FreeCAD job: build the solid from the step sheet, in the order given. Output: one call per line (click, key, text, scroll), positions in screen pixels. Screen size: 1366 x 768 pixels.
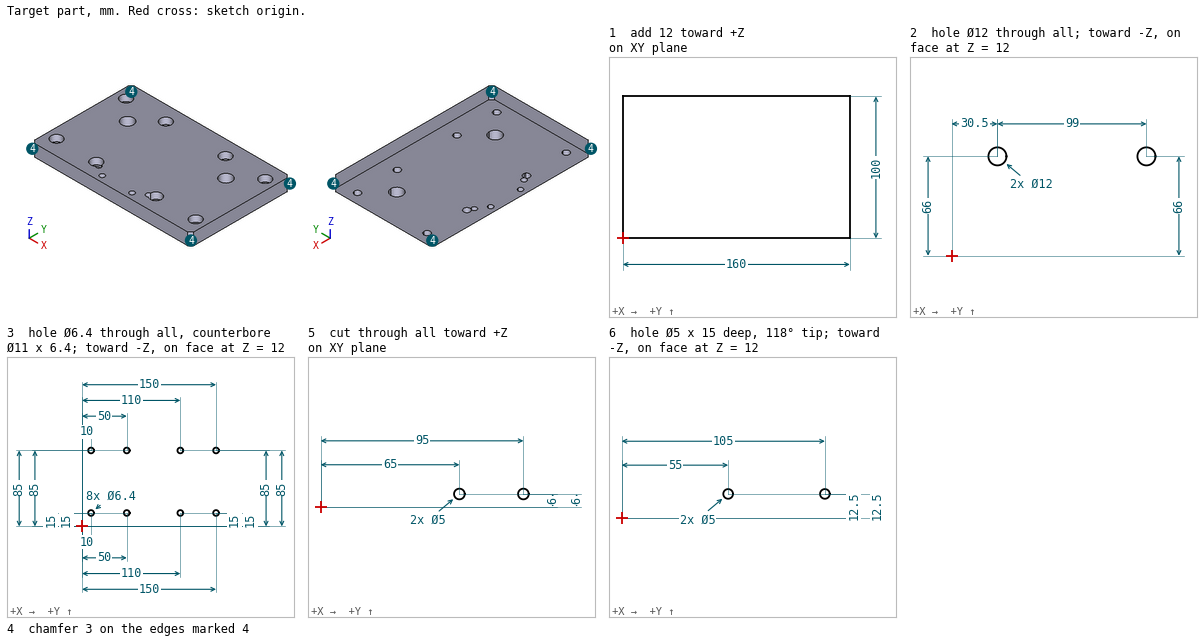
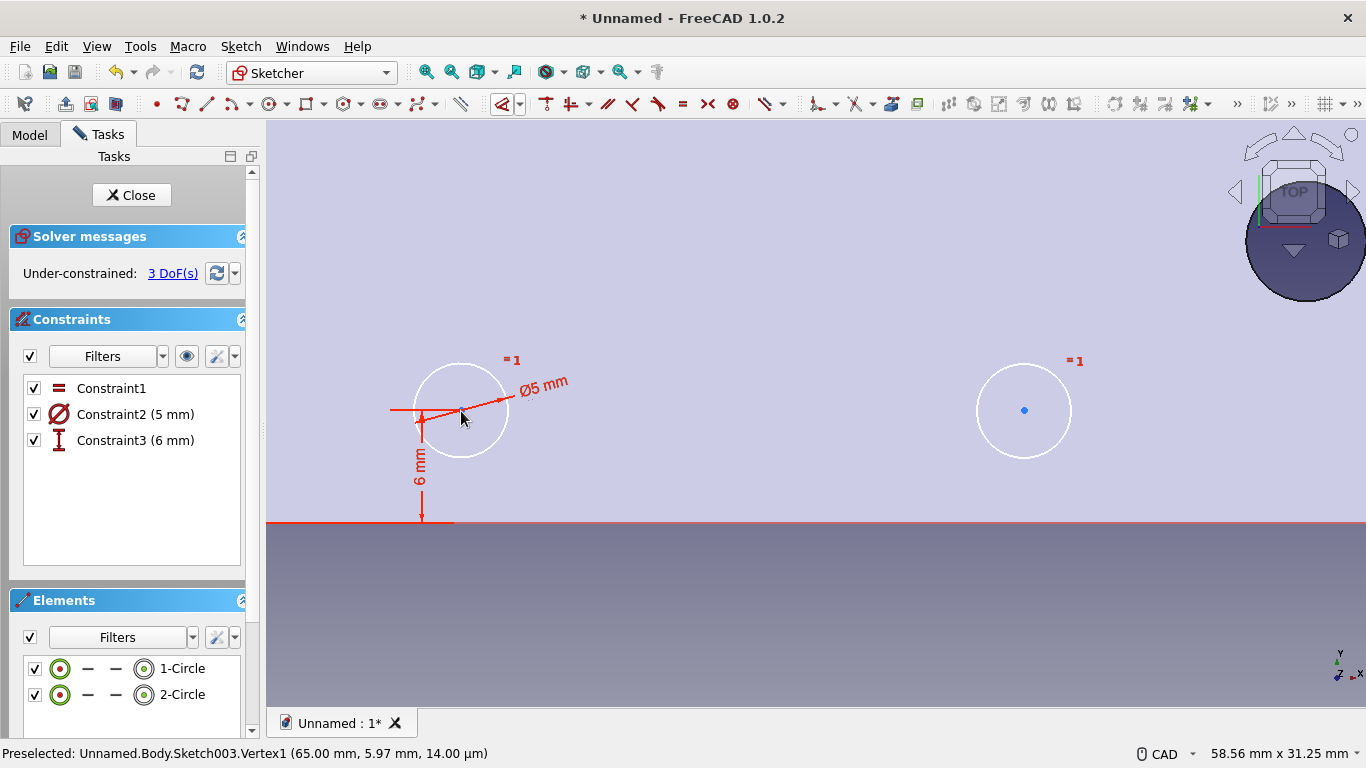
click(1024, 411)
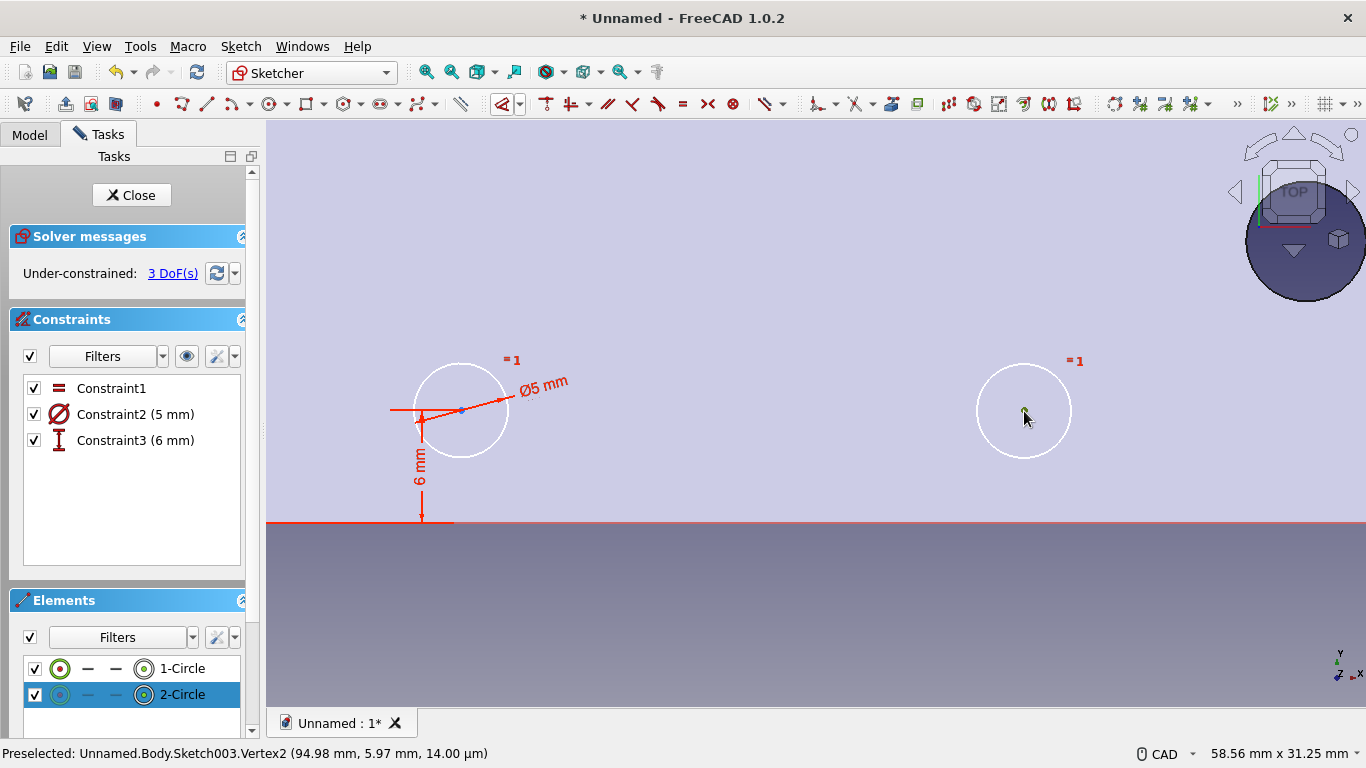
key(i)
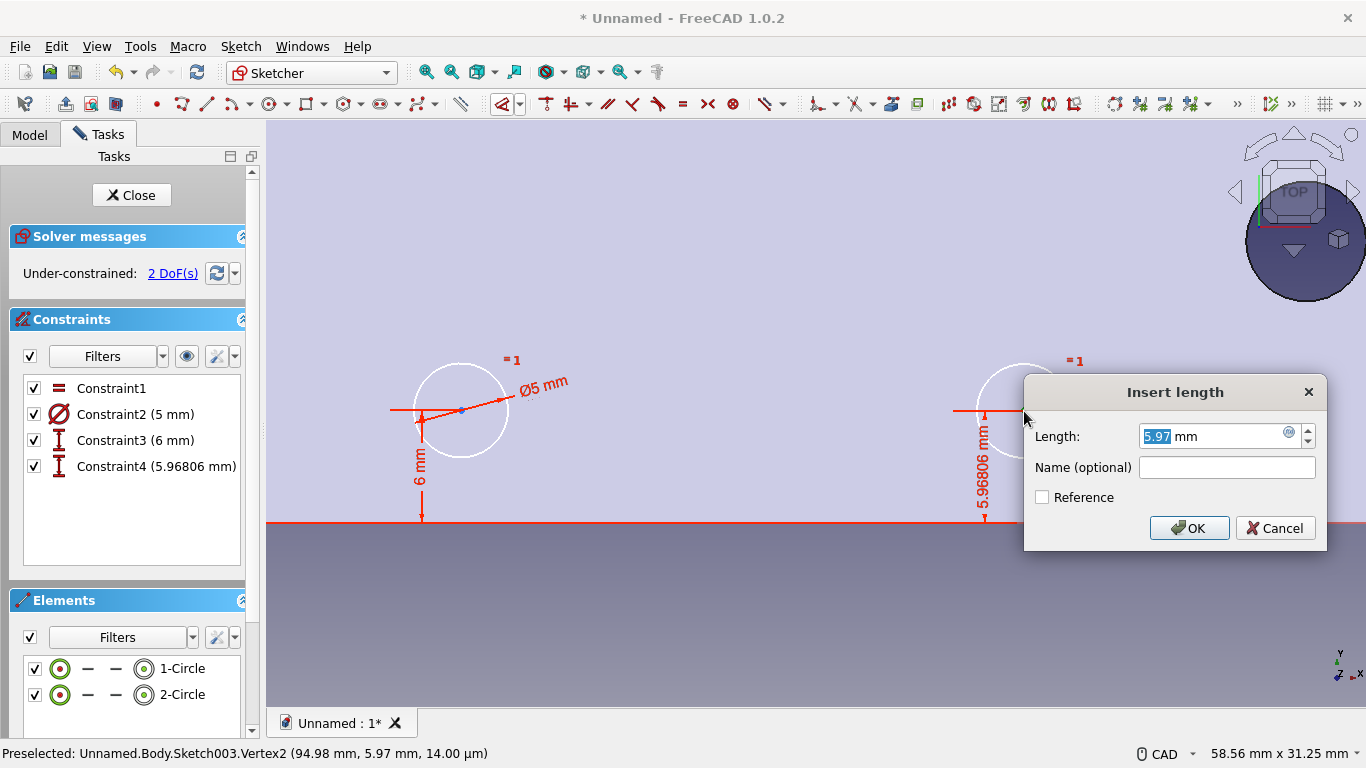
text(6)
key(Return)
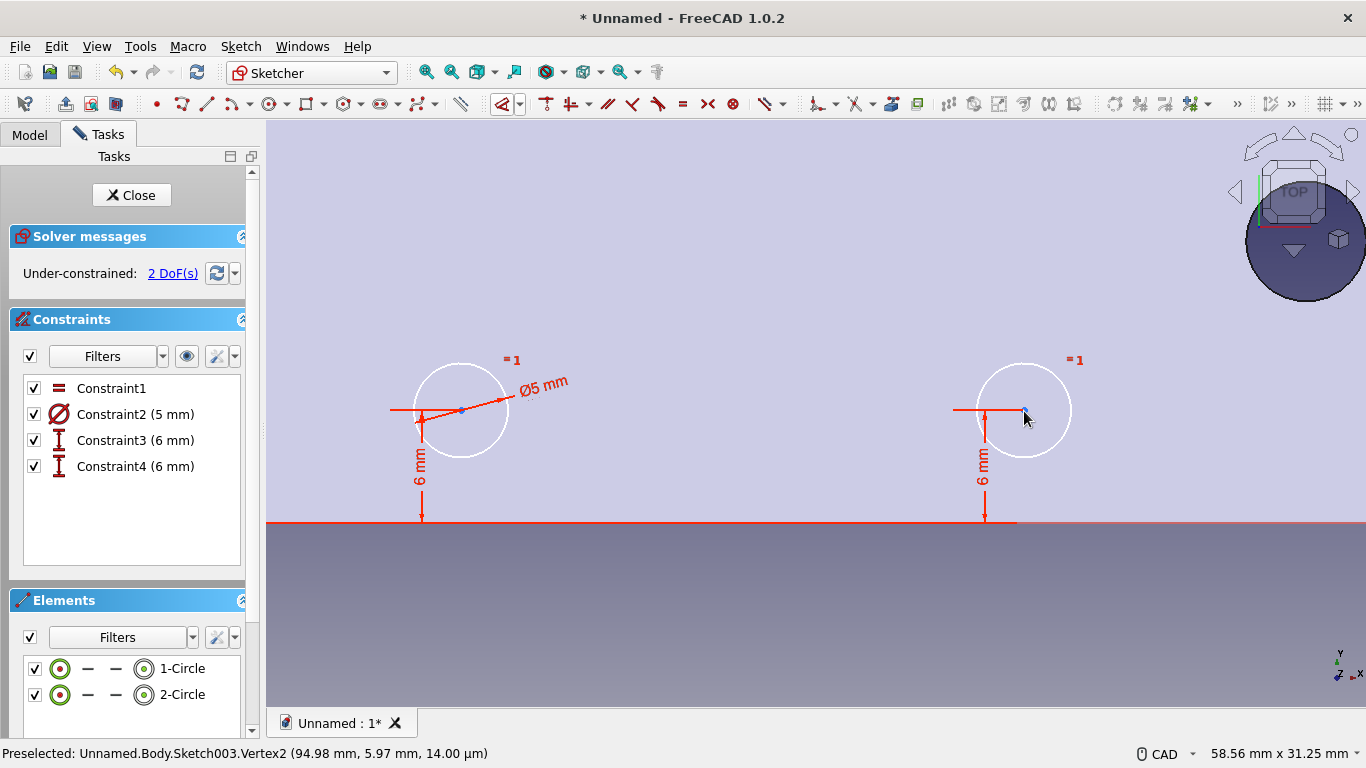
click(461, 410)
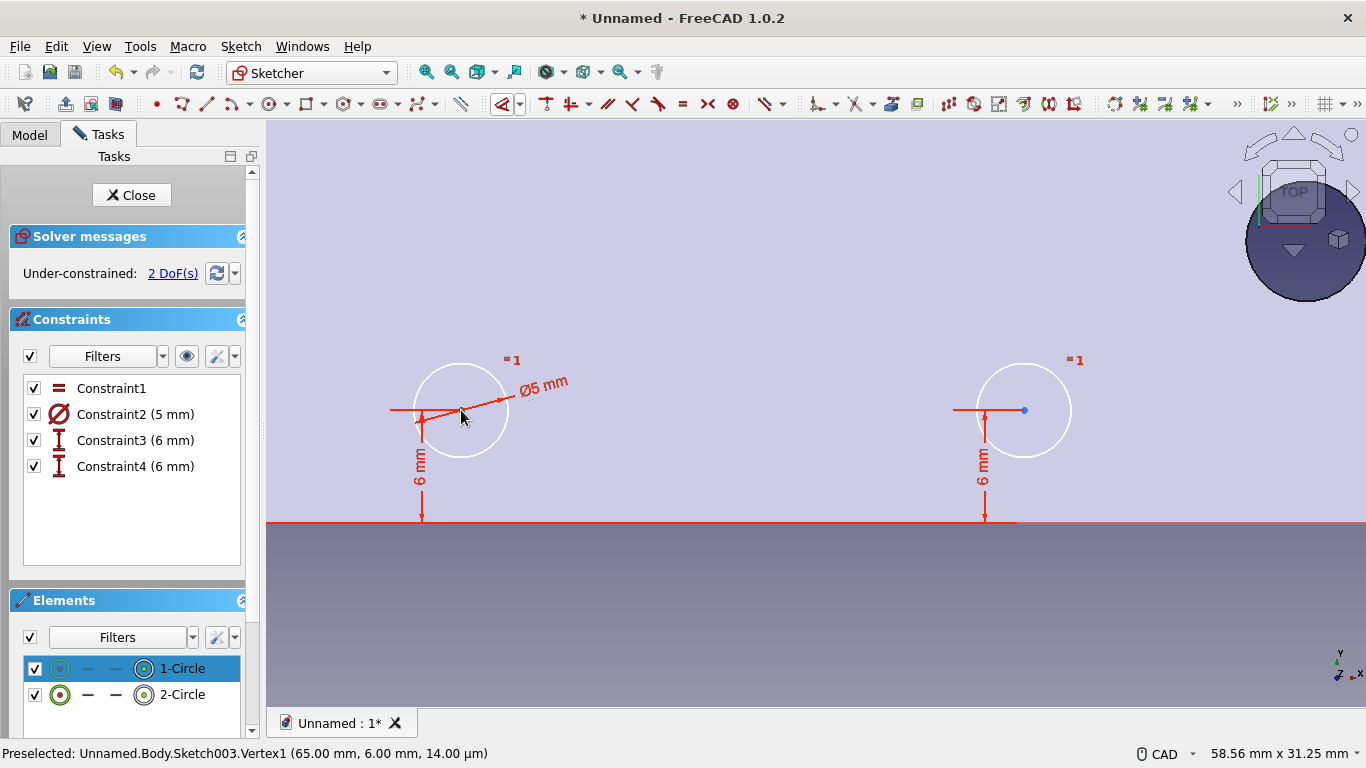
key(l)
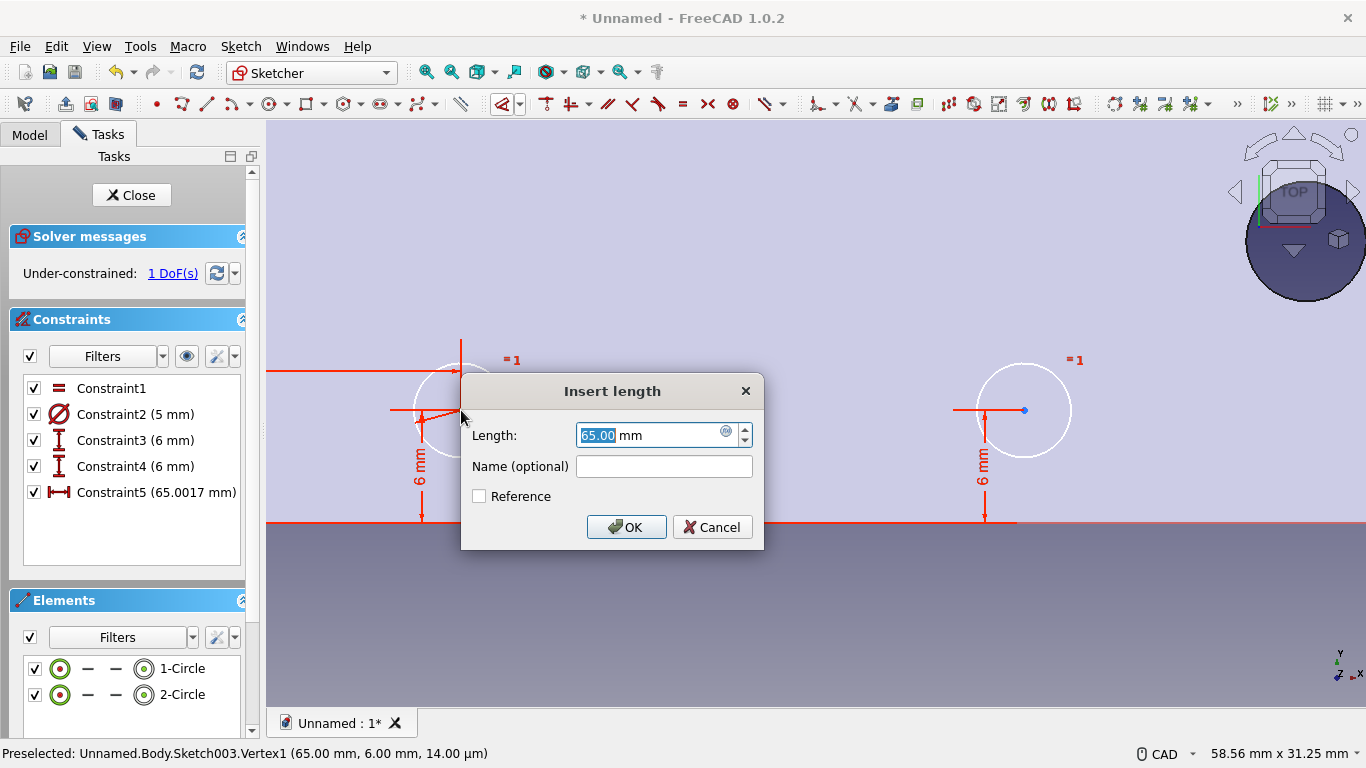
text(65)
key(Return)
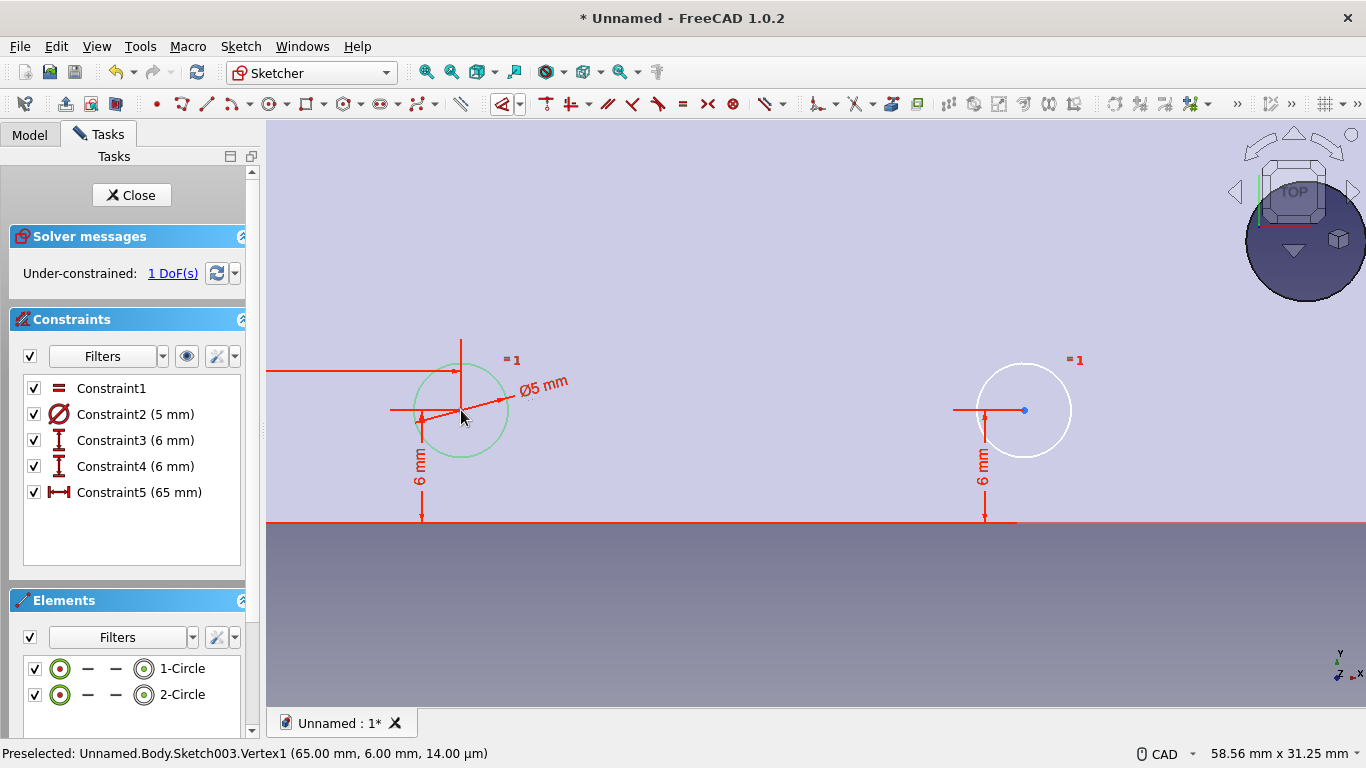
click(1024, 410)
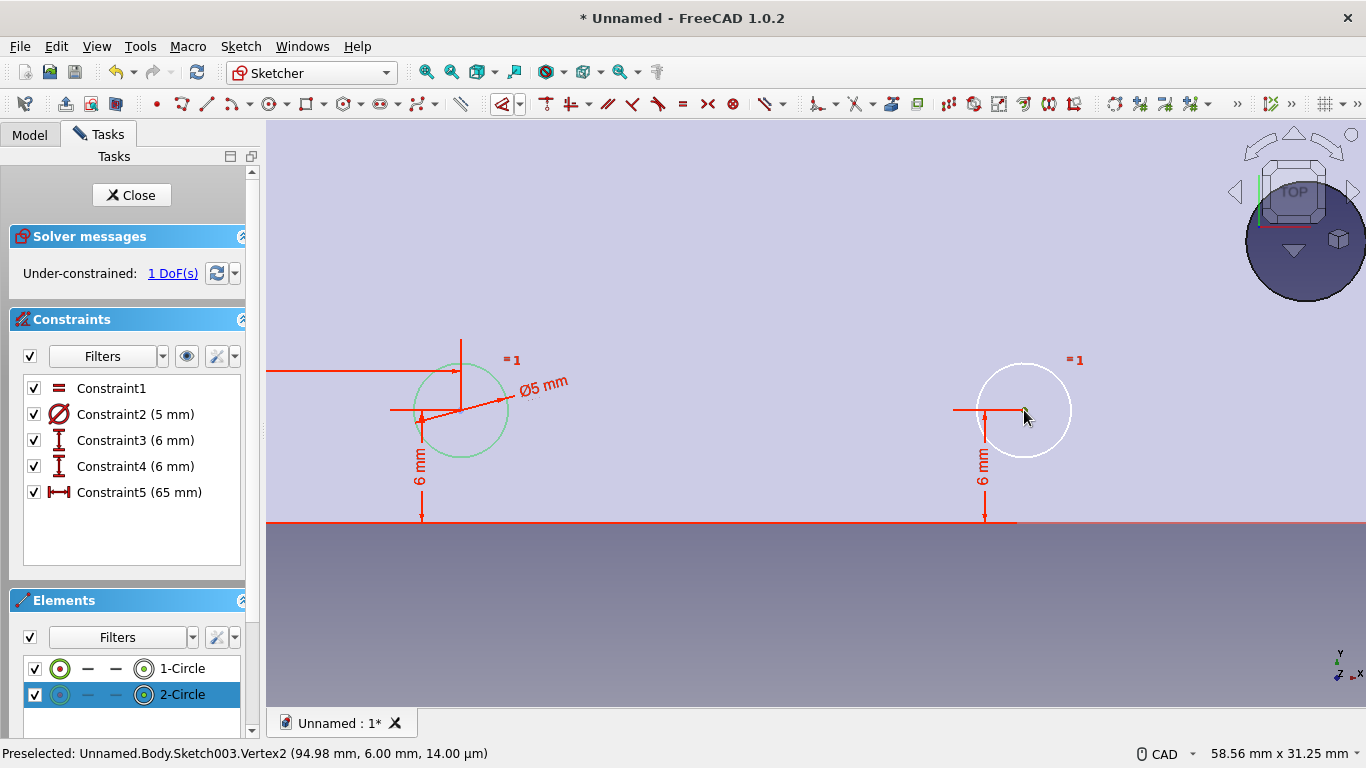
key(l)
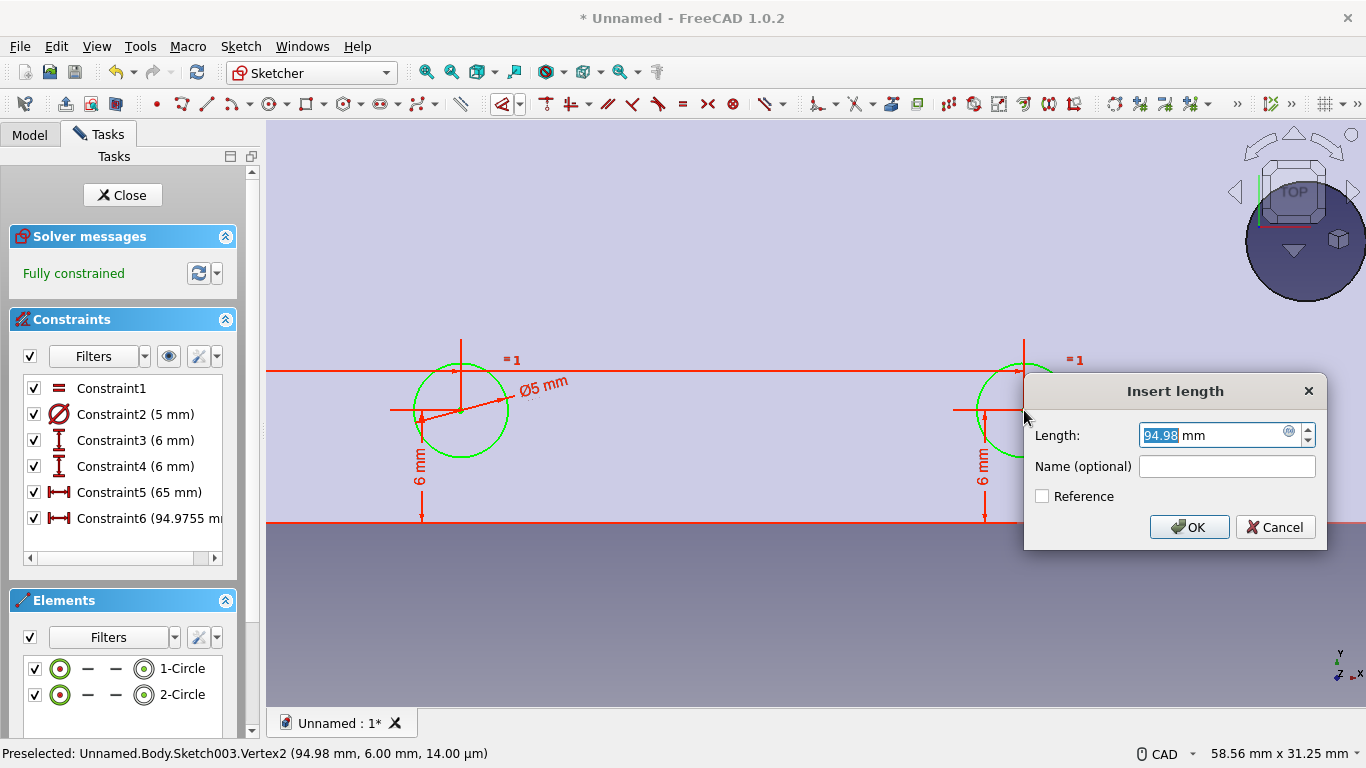
text(95)
key(Return)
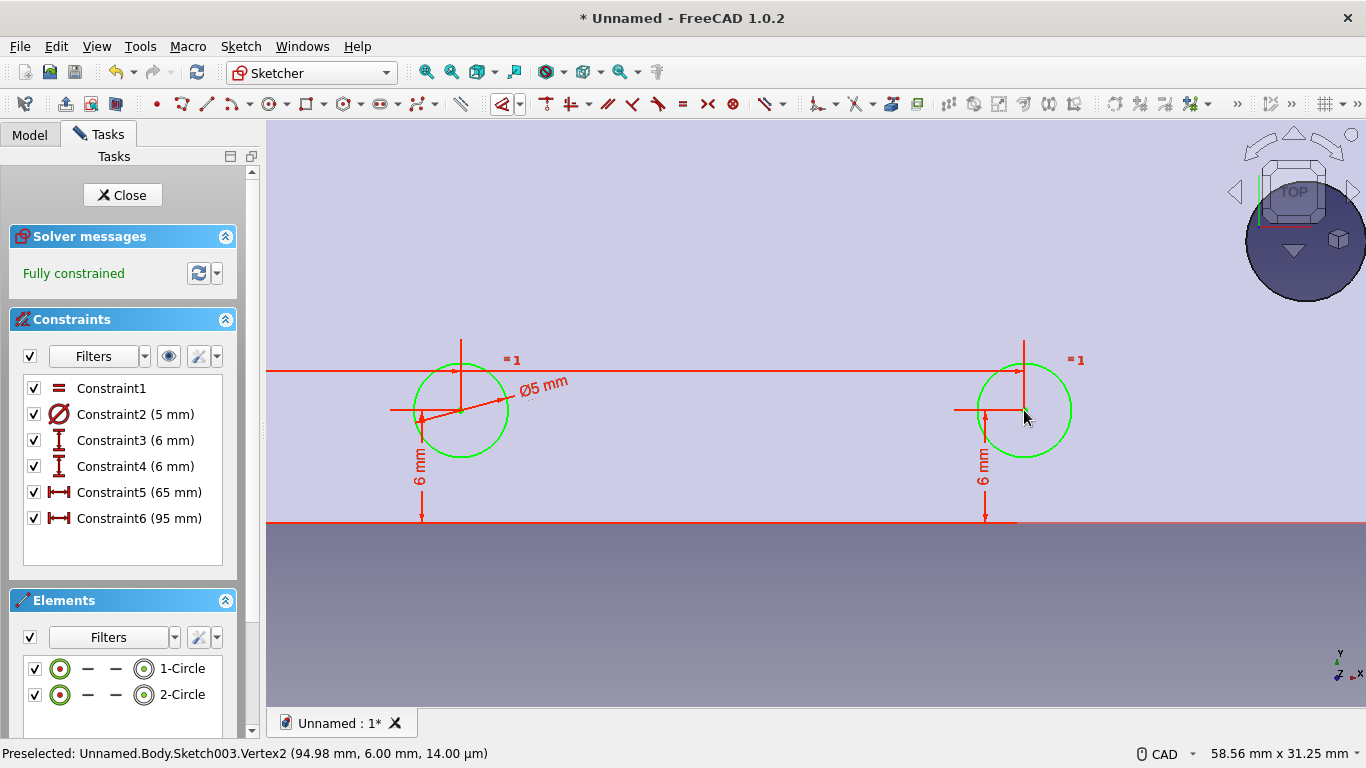
click(123, 195)